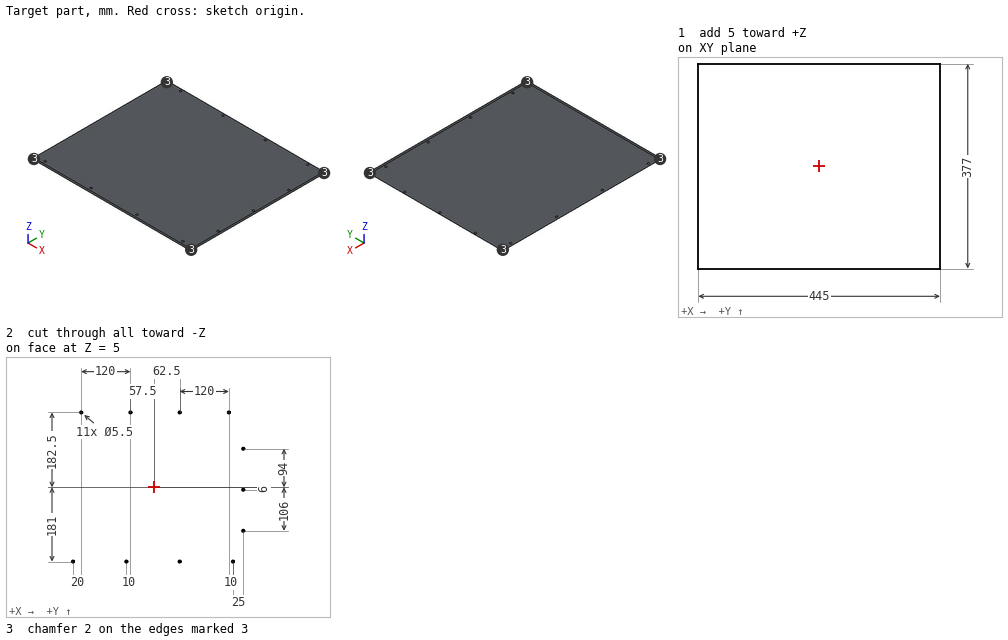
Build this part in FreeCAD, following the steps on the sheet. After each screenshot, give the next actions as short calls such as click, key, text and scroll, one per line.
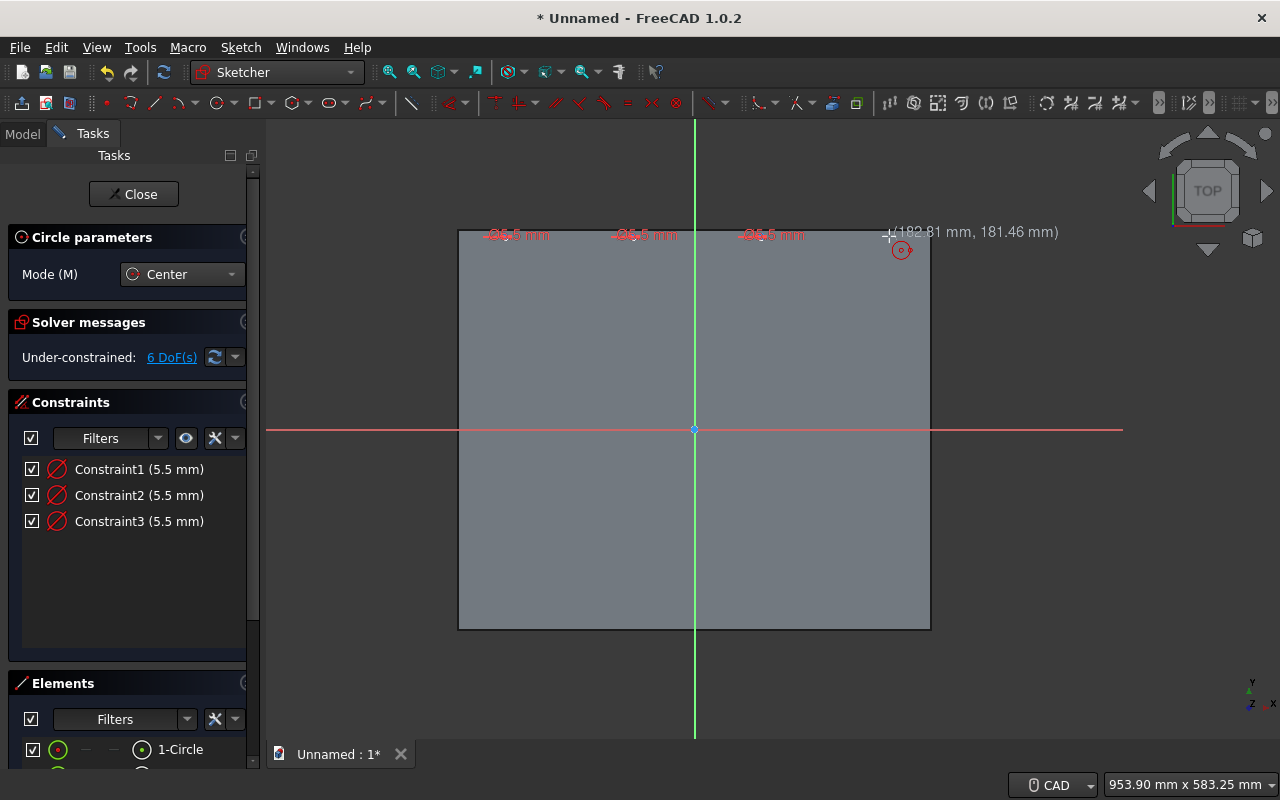
click(889, 236)
move(891, 234)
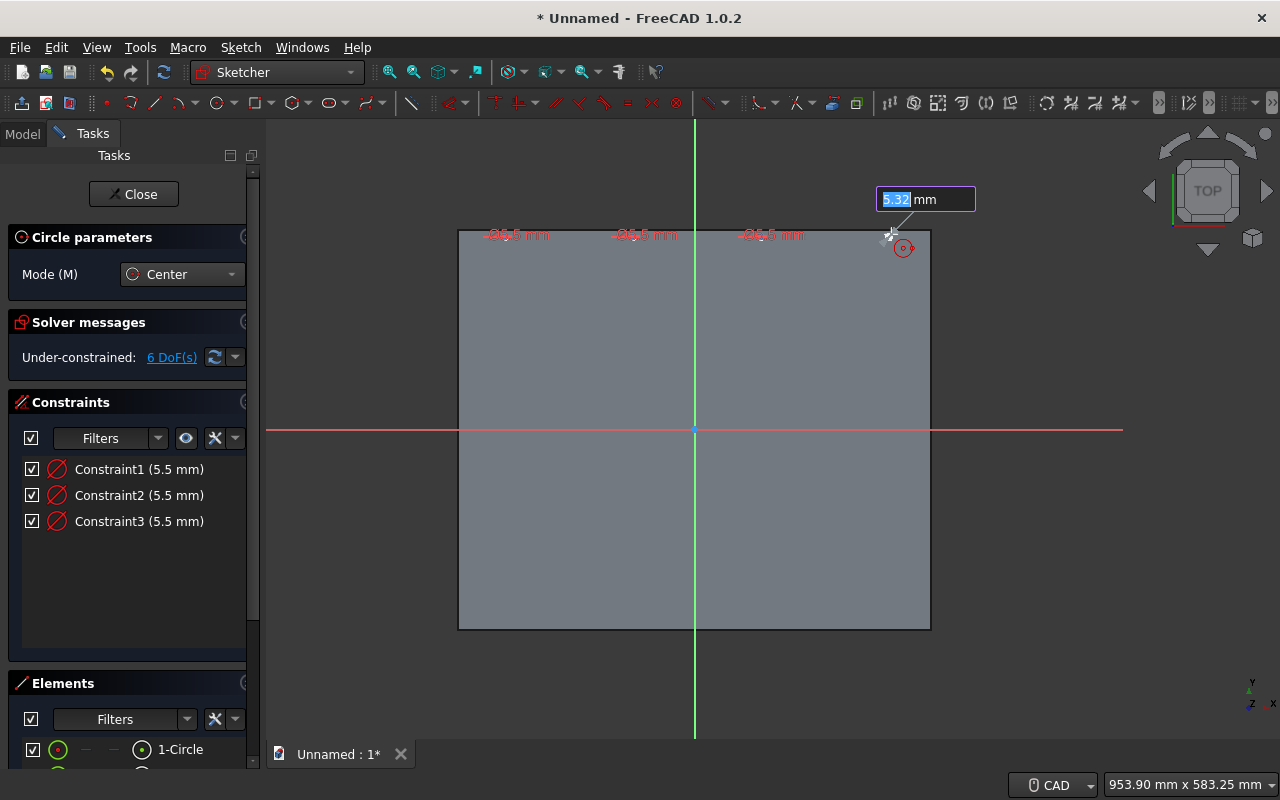
text(5.5)
key(Return)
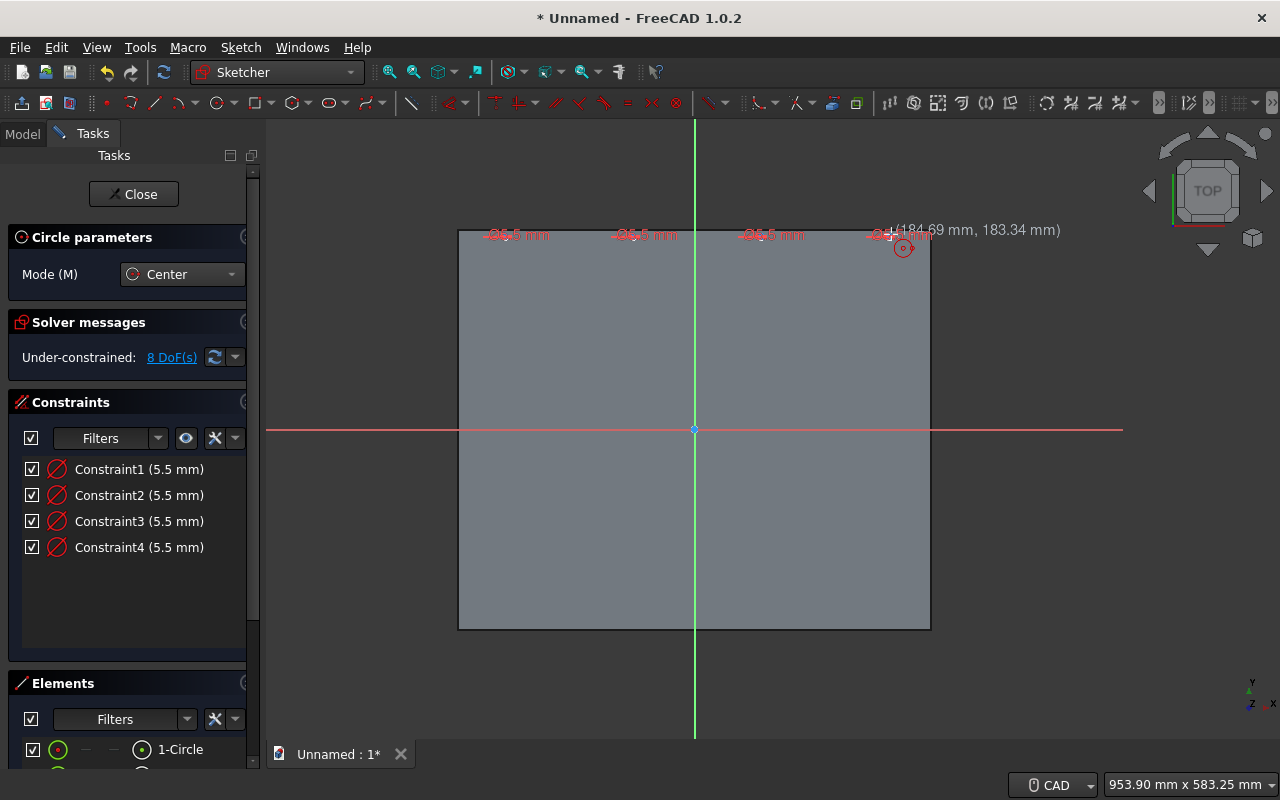
scroll(485, 622, up, 11)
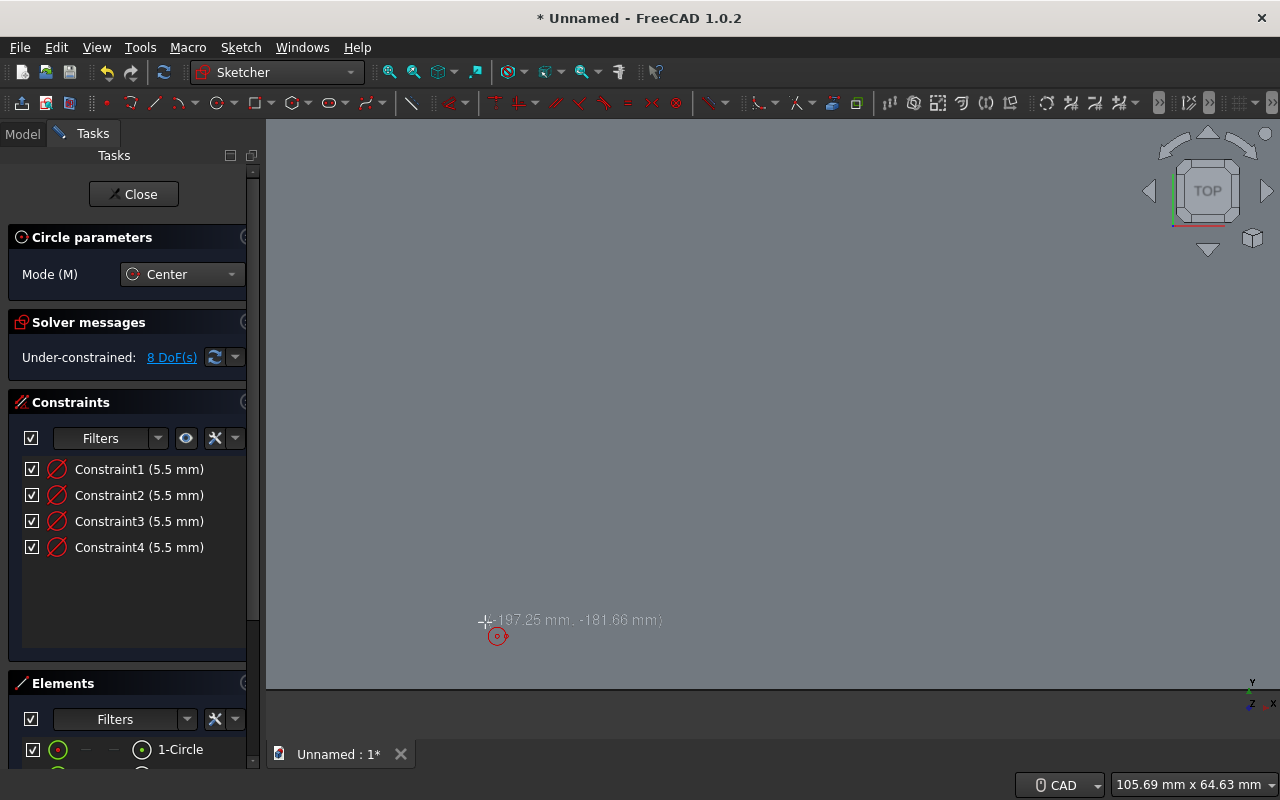
scroll(484, 623, down, 11)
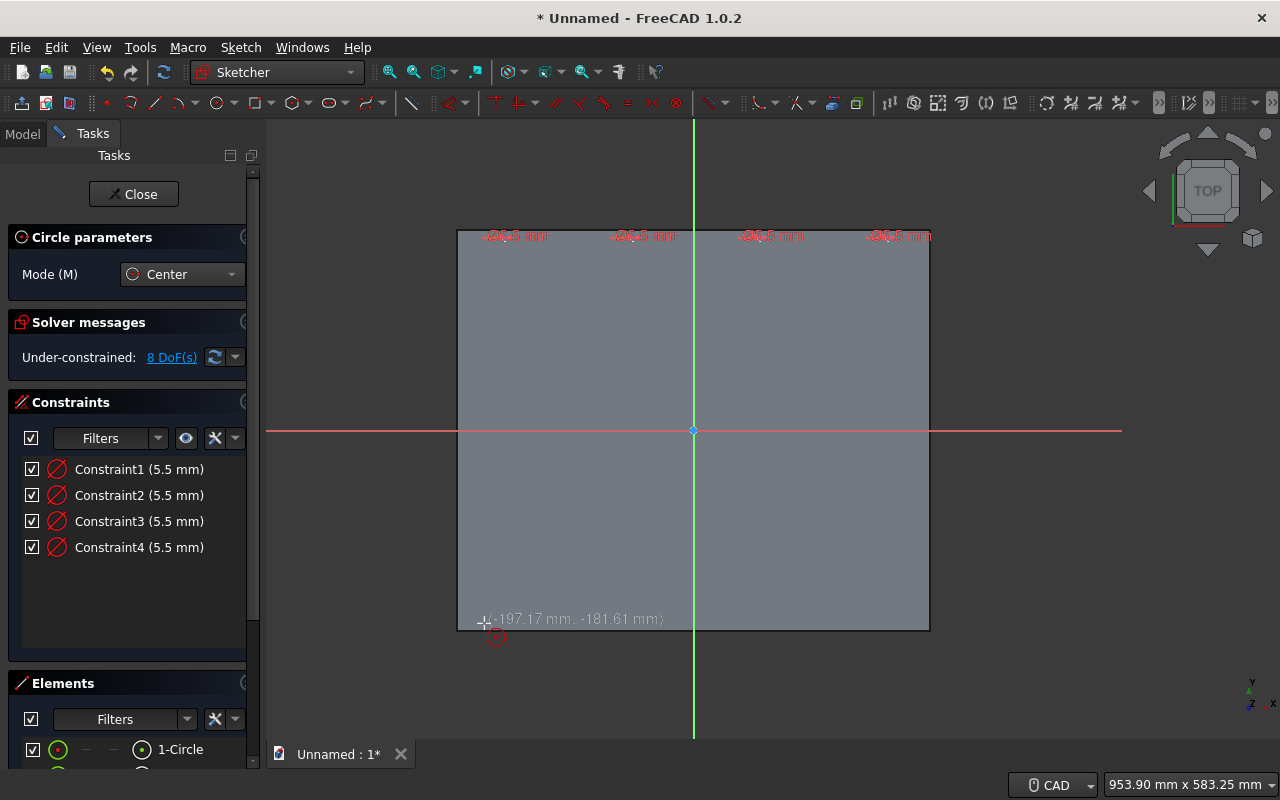
click(484, 623)
move(486, 621)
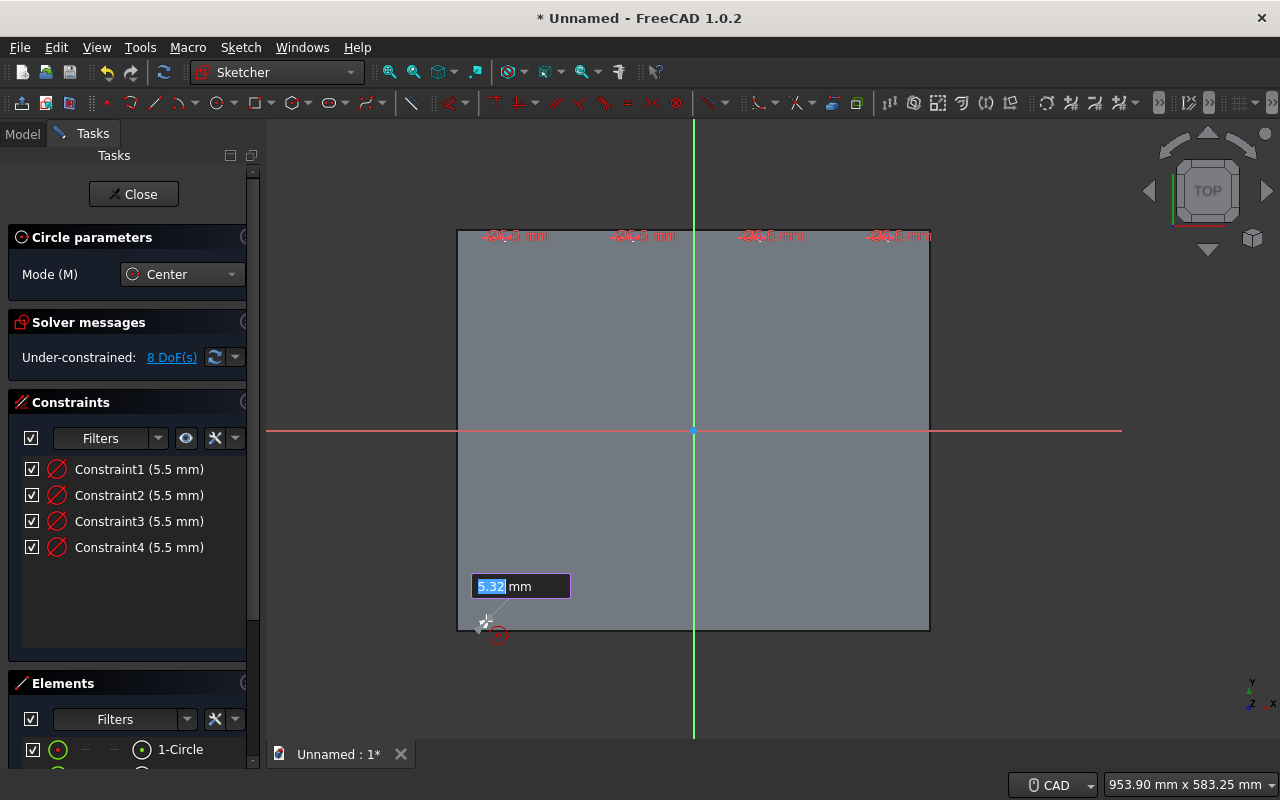
text(5.5)
key(Return)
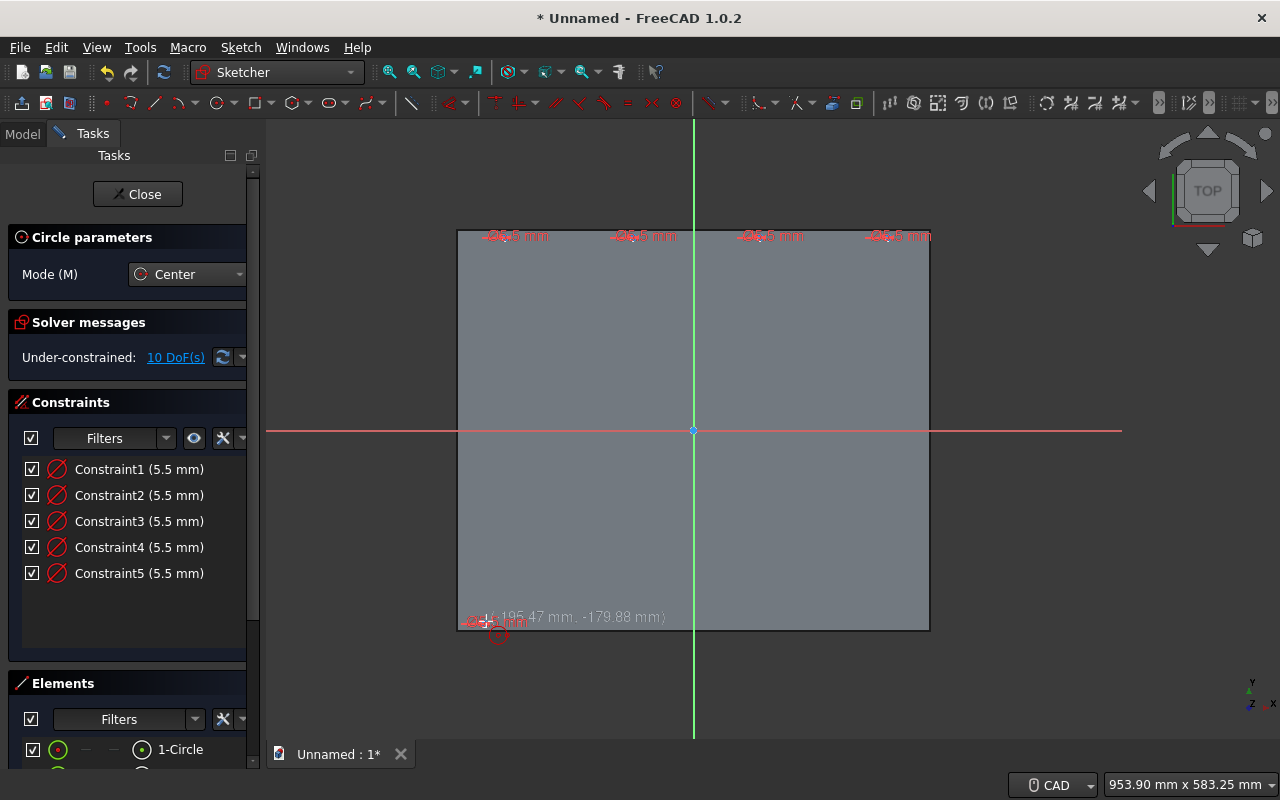
scroll(622, 623, up, 11)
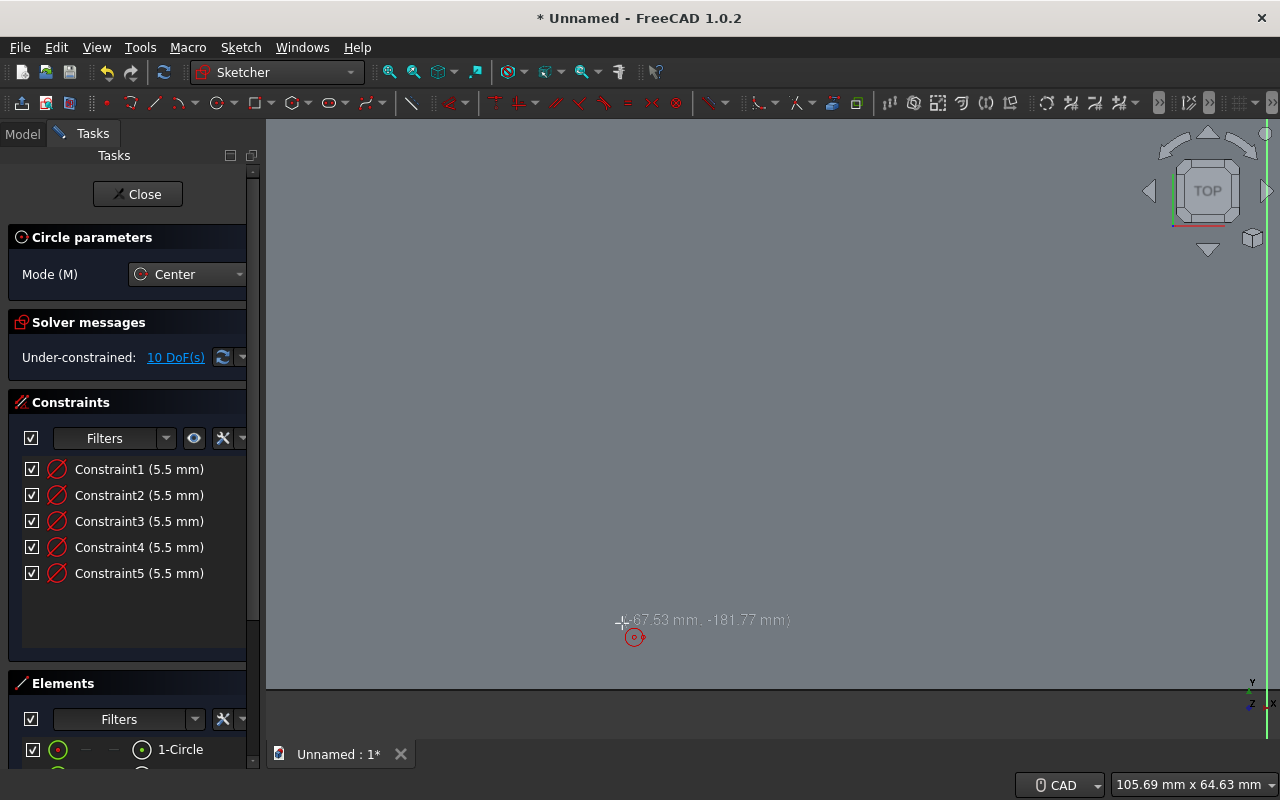
scroll(622, 623, down, 11)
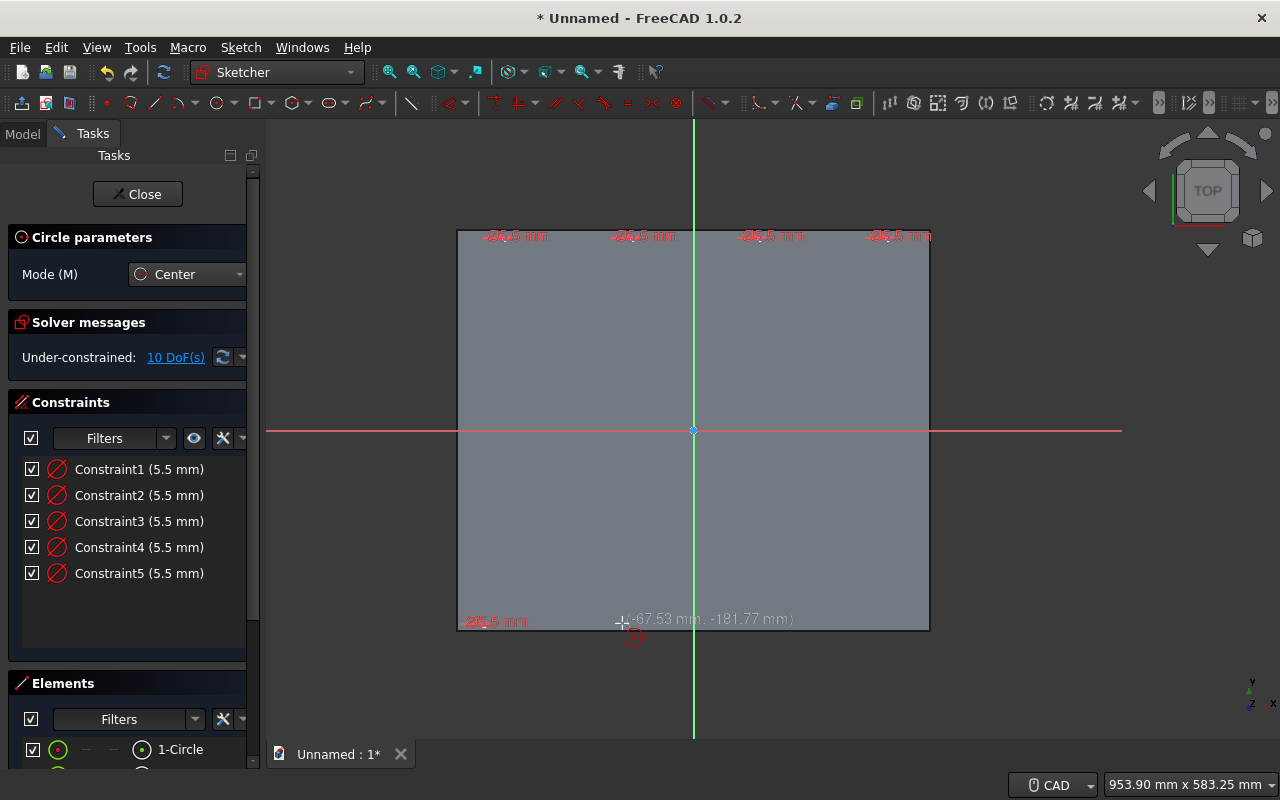
click(622, 623)
move(624, 621)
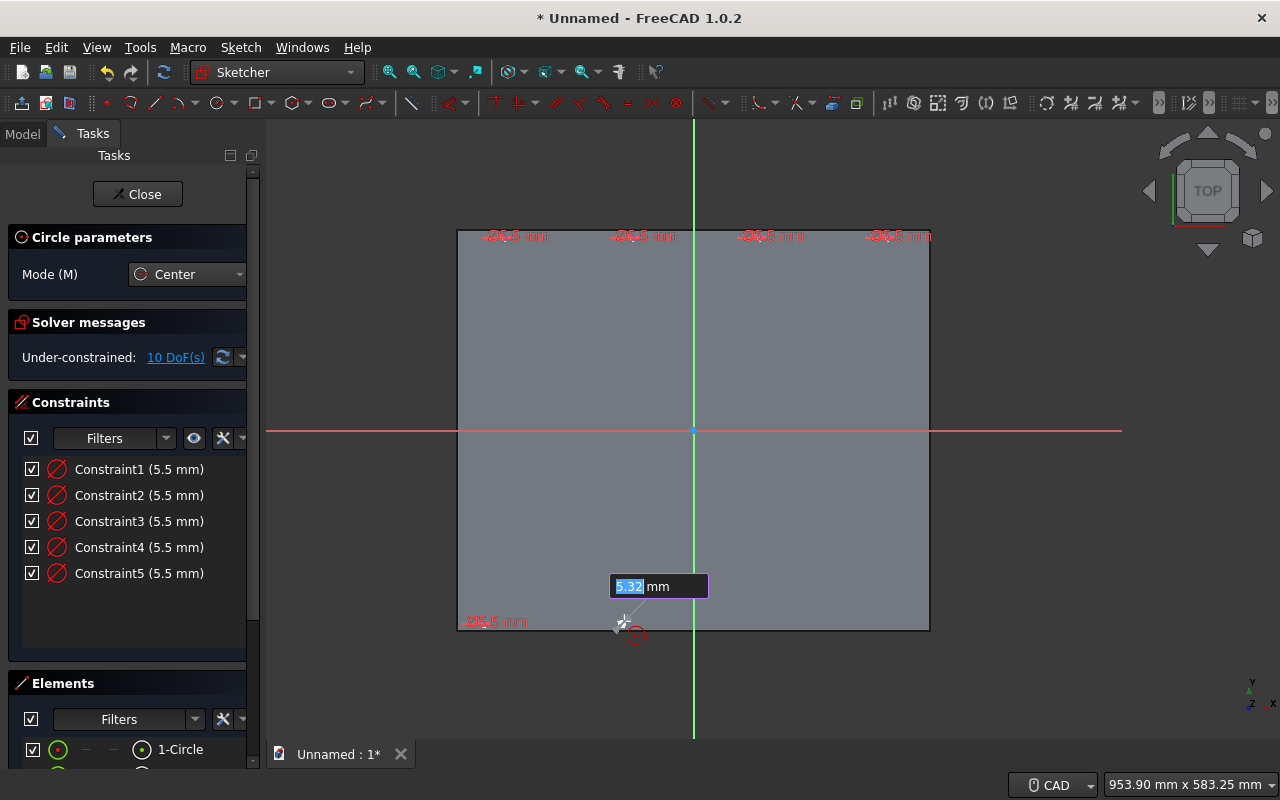
text(5.5)
key(Return)